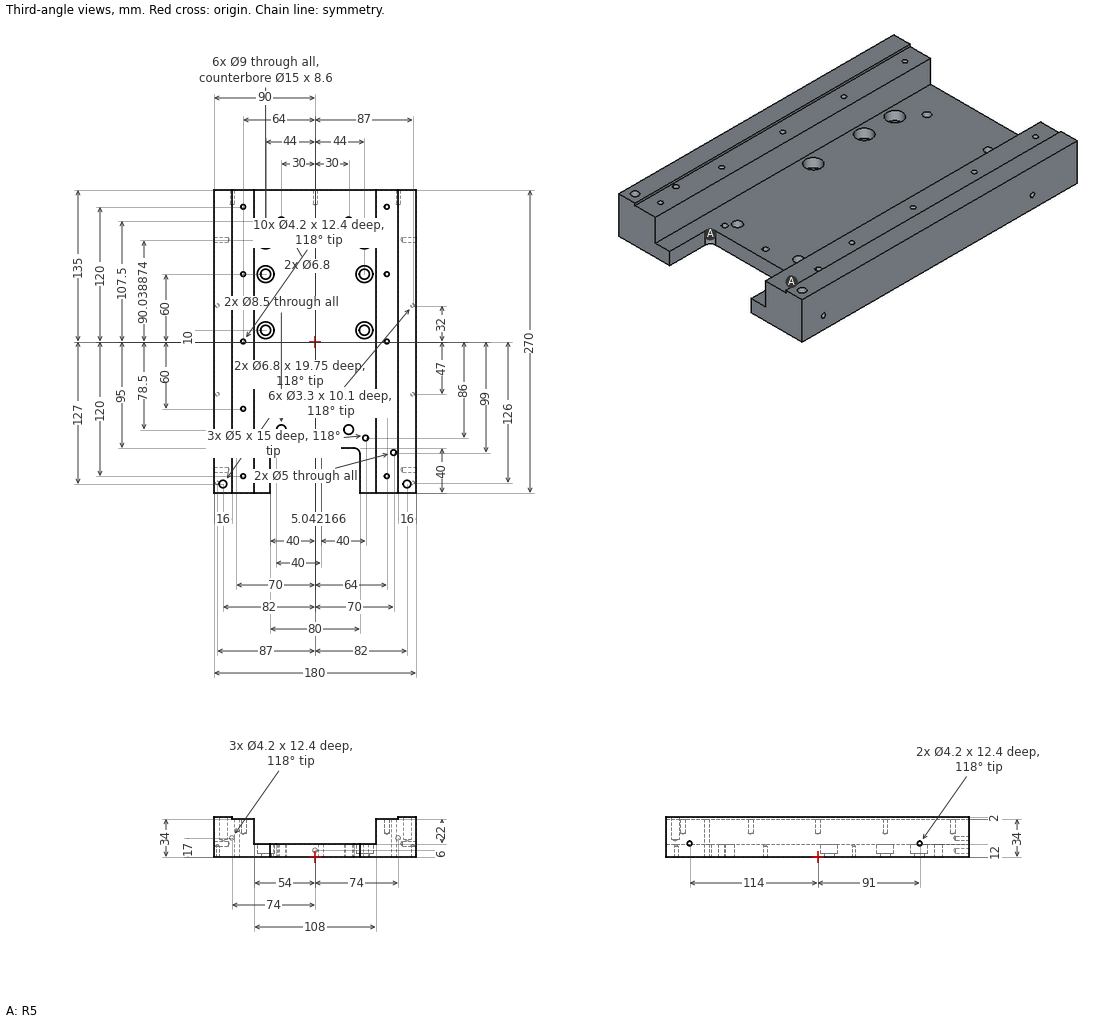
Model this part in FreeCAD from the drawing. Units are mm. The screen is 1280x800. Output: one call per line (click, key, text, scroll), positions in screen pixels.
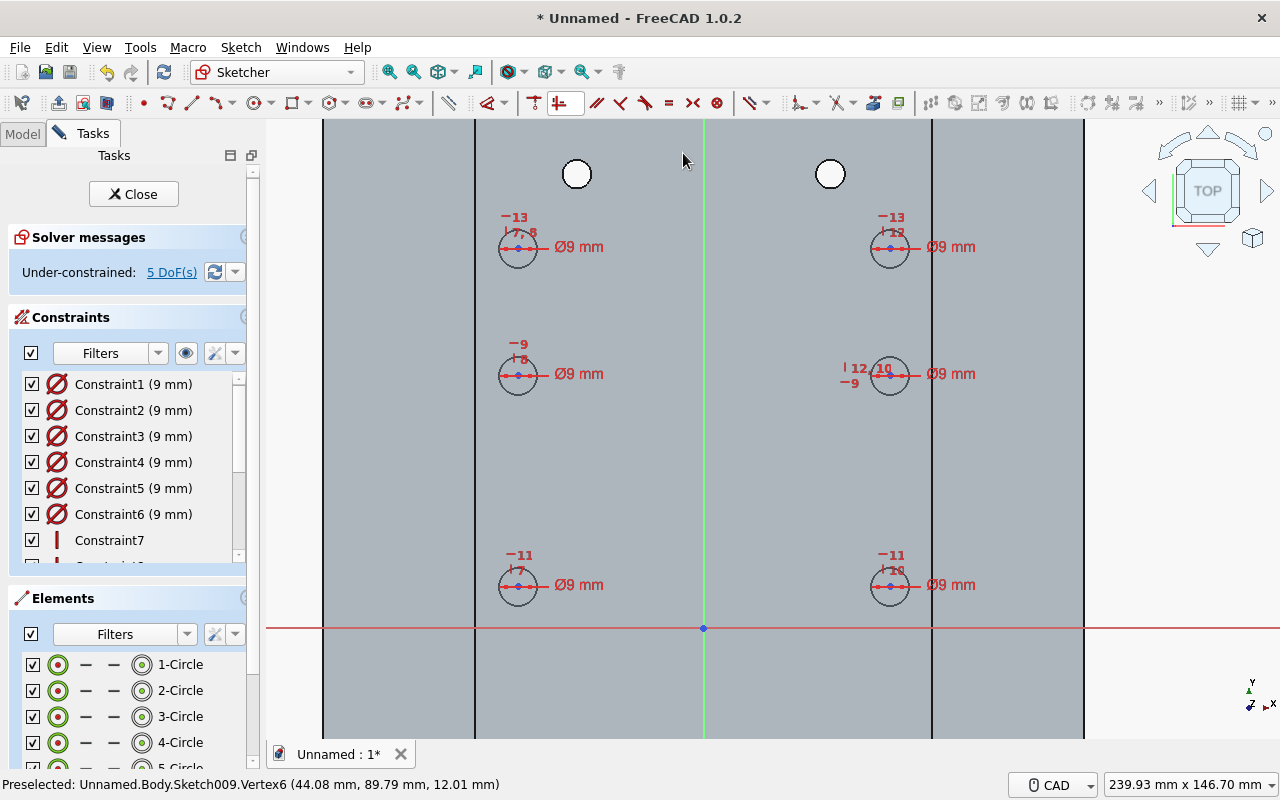
click(488, 104)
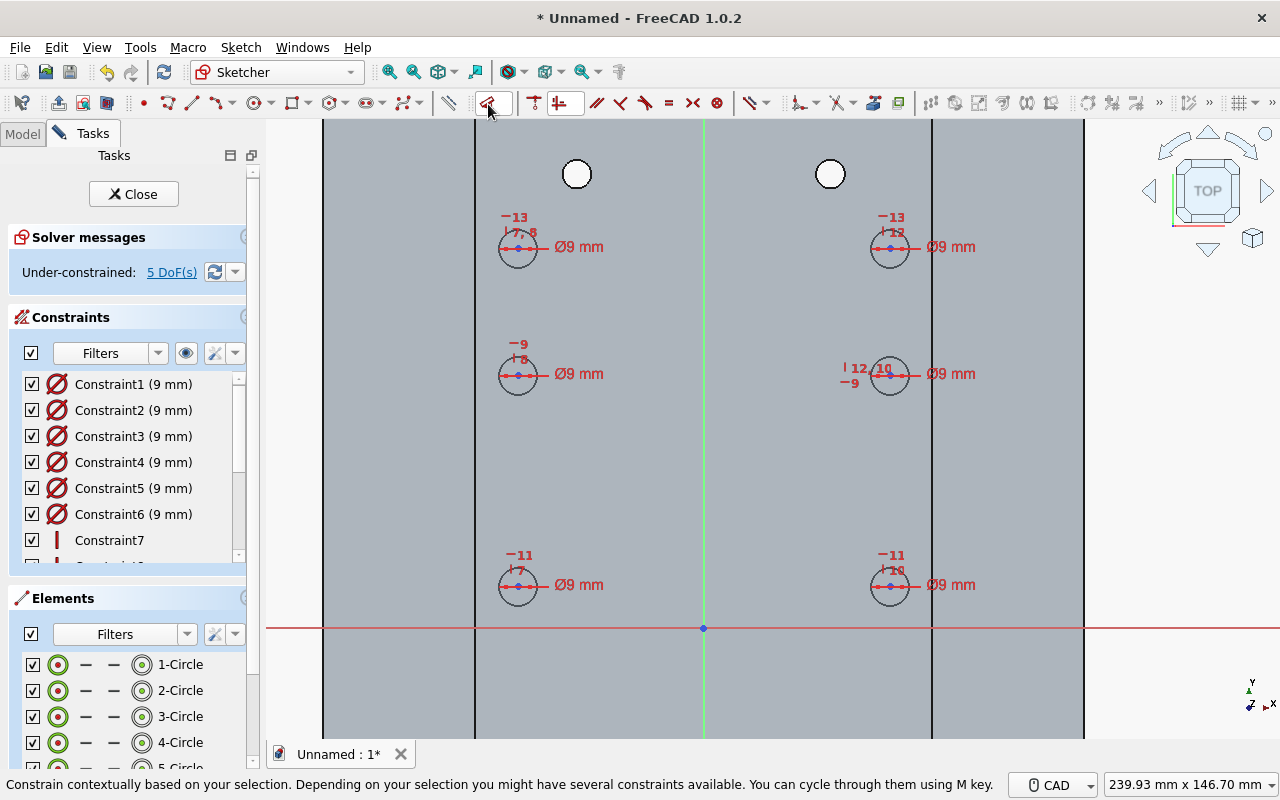
click(518, 249)
click(611, 662)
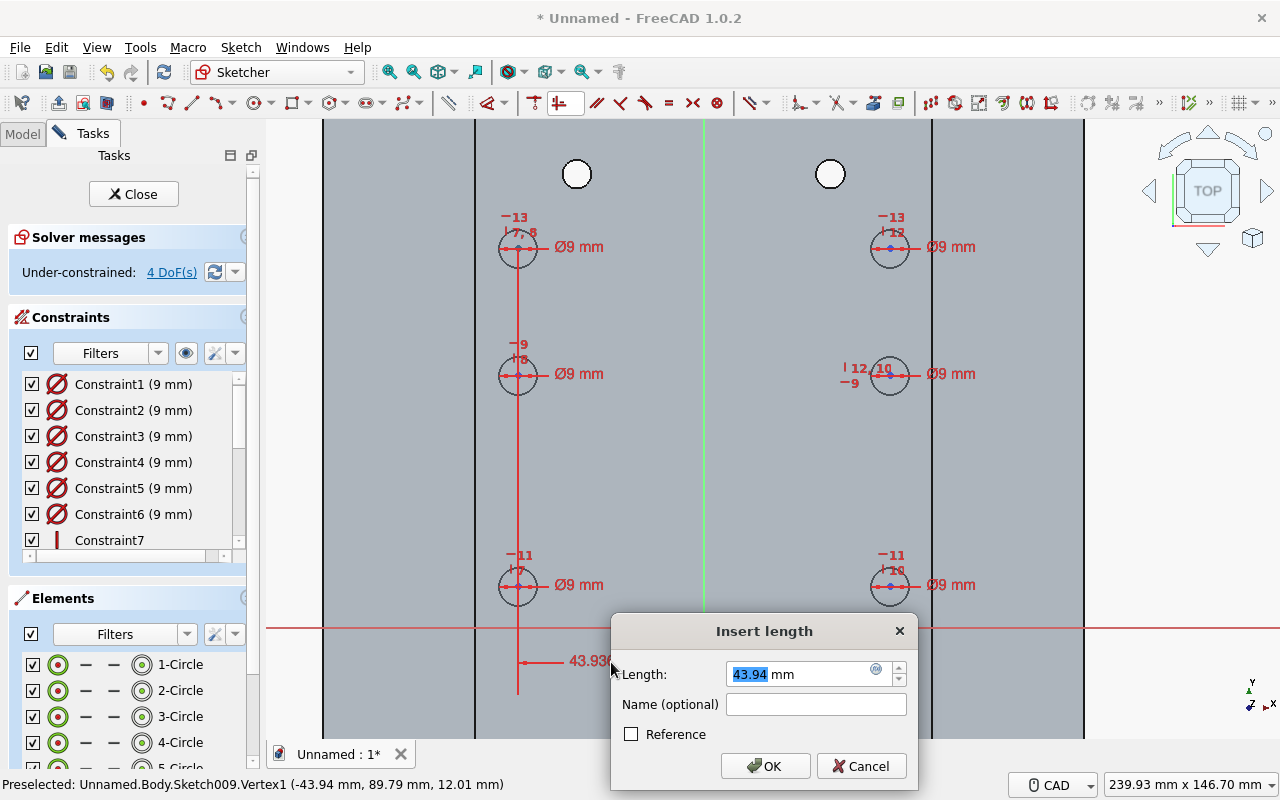
text(44)
key(Return)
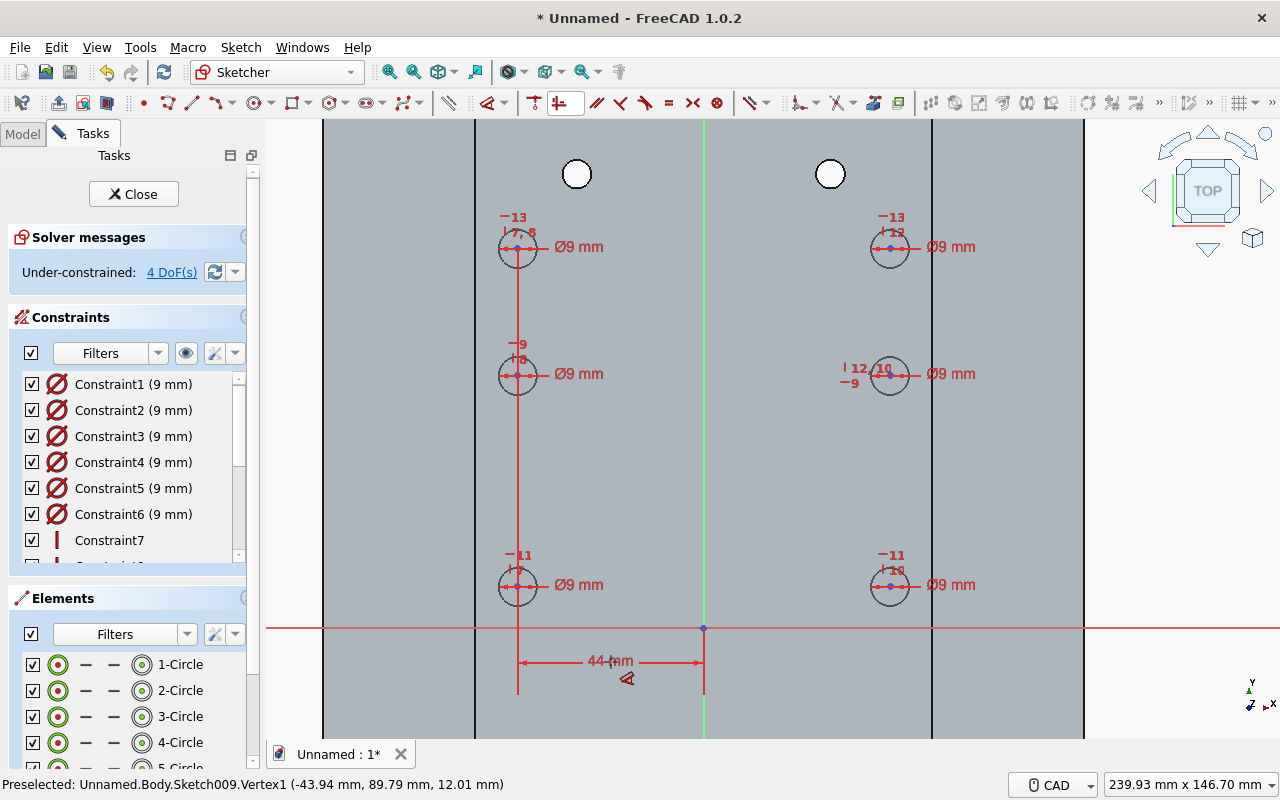
click(518, 587)
click(484, 608)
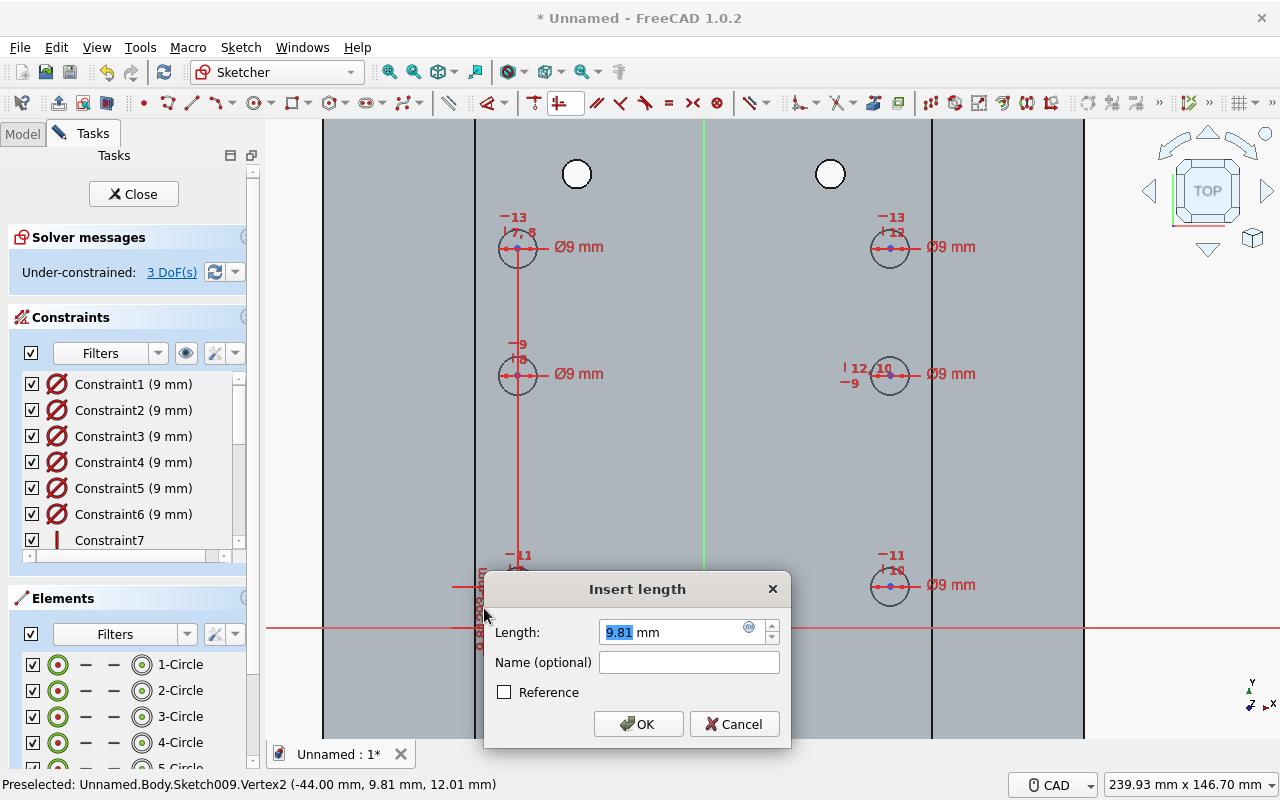
text(10)
key(Return)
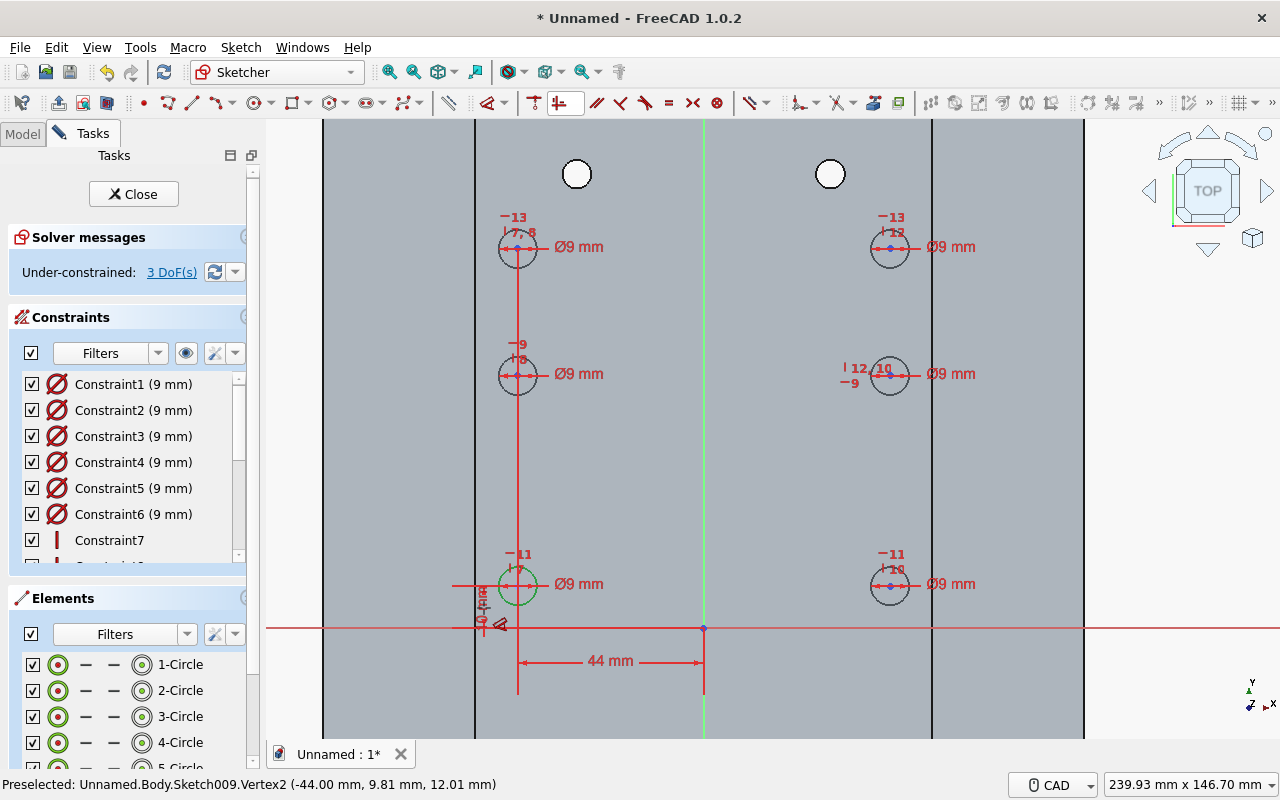
click(518, 376)
click(484, 502)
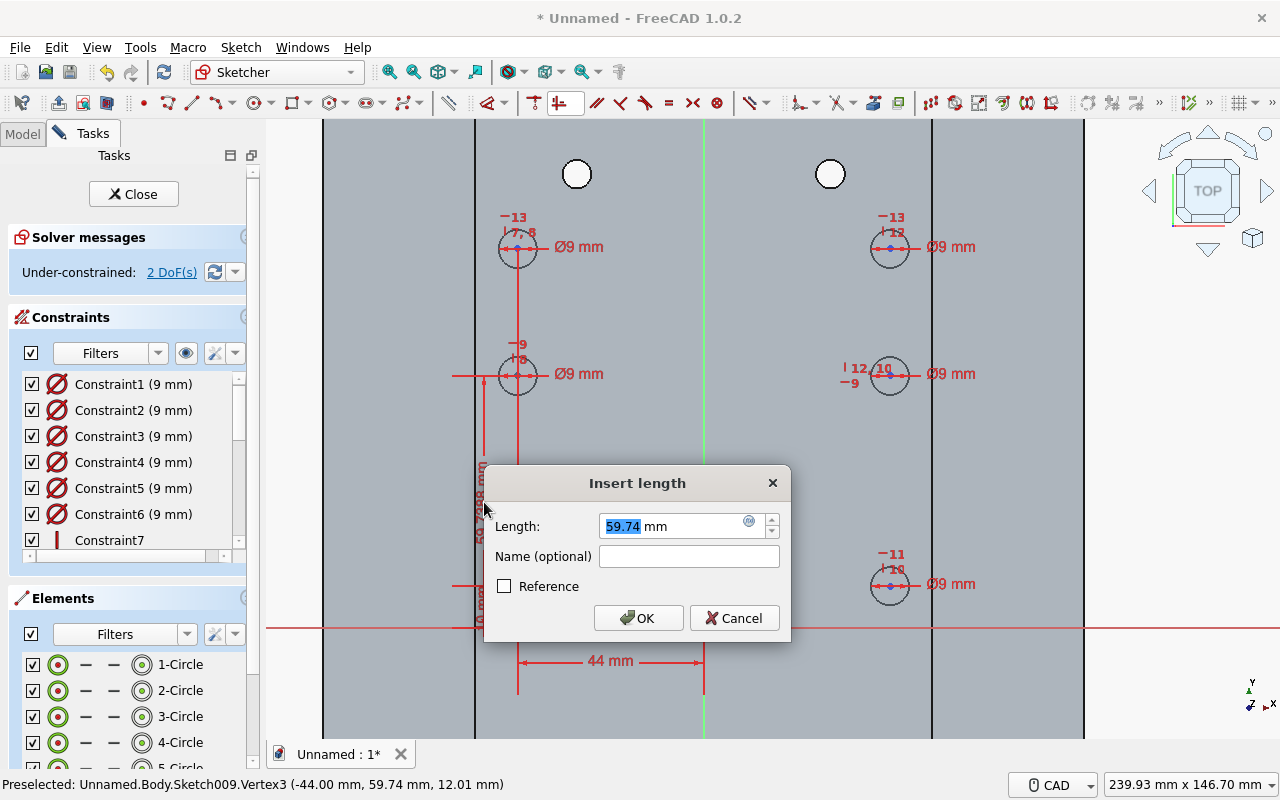
text(60)
key(Return)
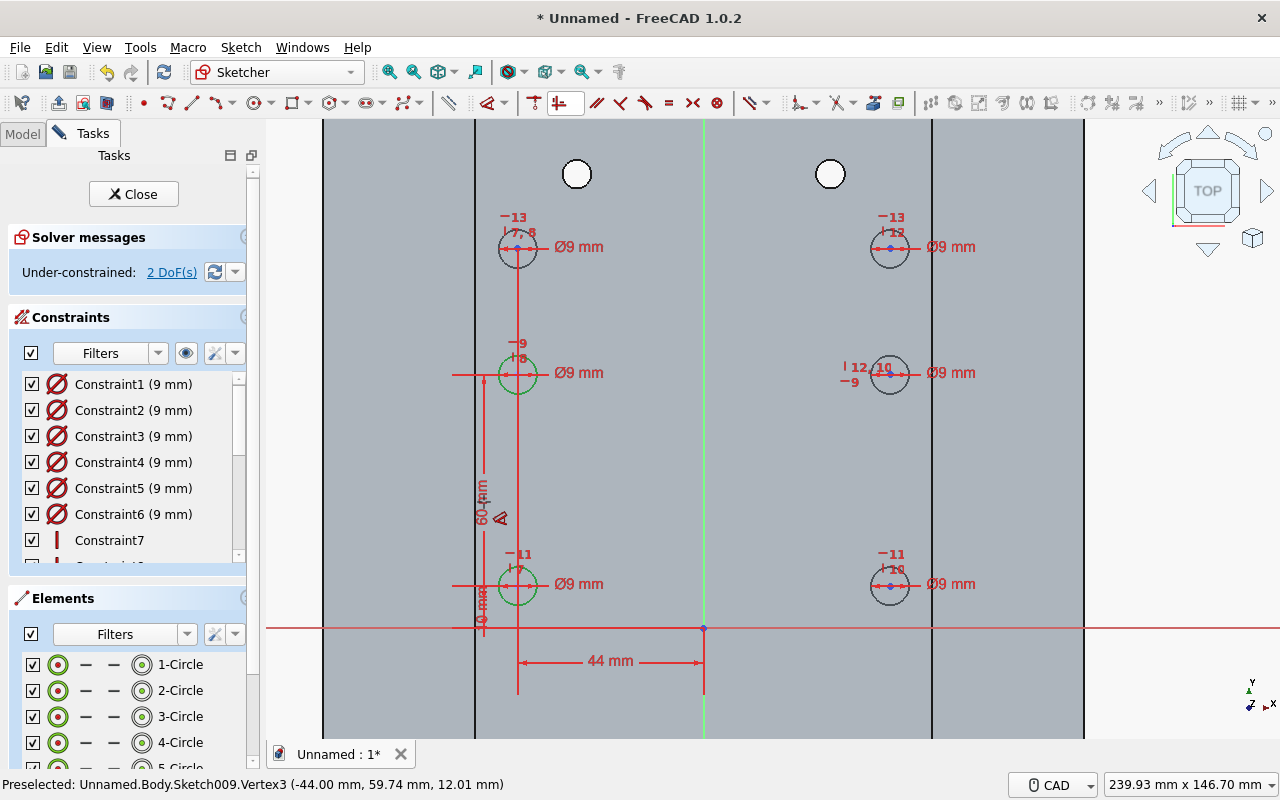
click(890, 375)
click(797, 662)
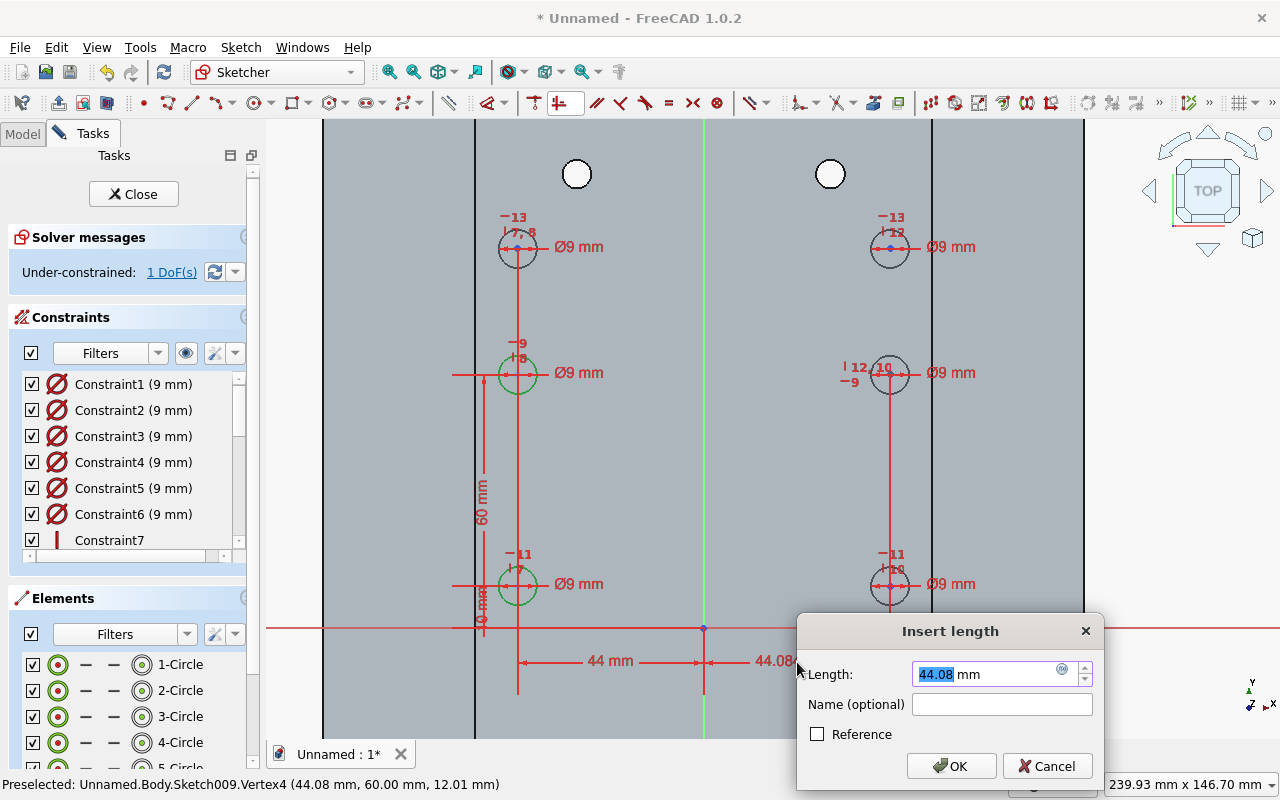
text(44)
key(Return)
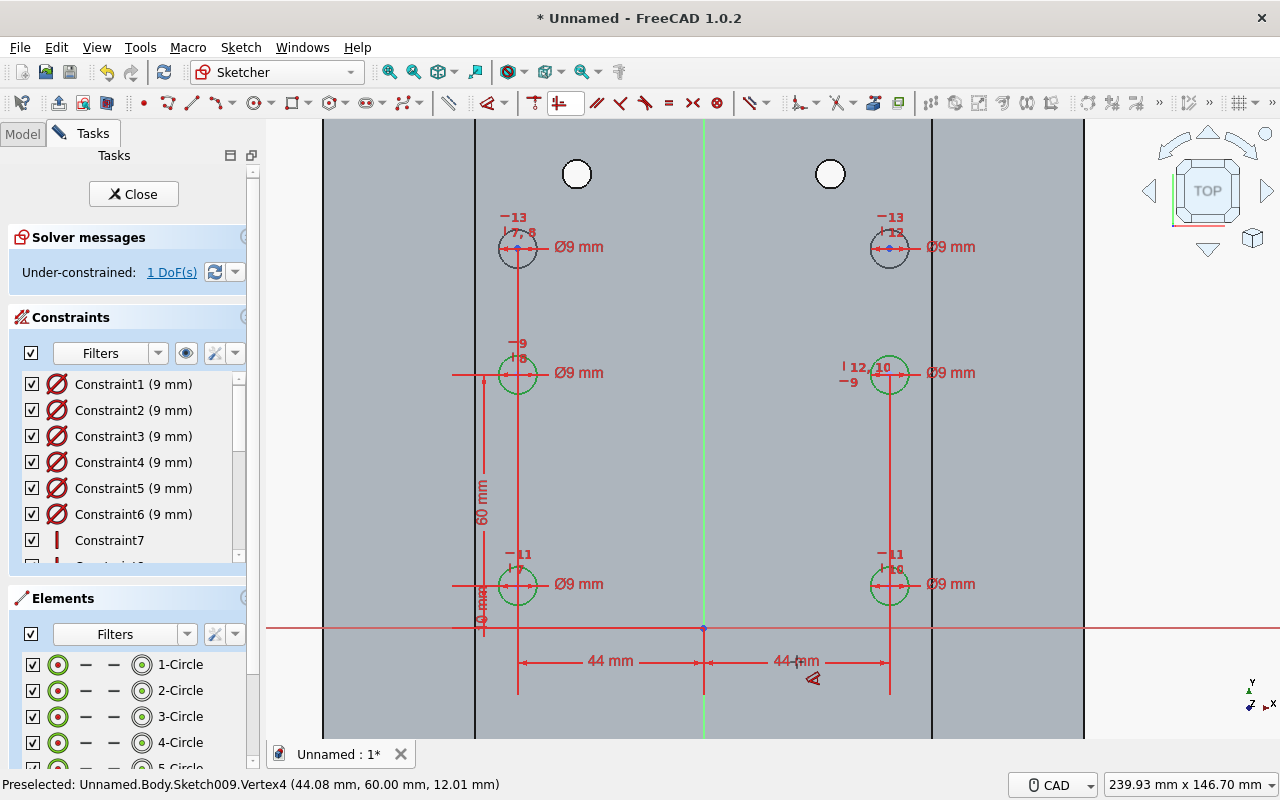
click(518, 249)
click(484, 439)